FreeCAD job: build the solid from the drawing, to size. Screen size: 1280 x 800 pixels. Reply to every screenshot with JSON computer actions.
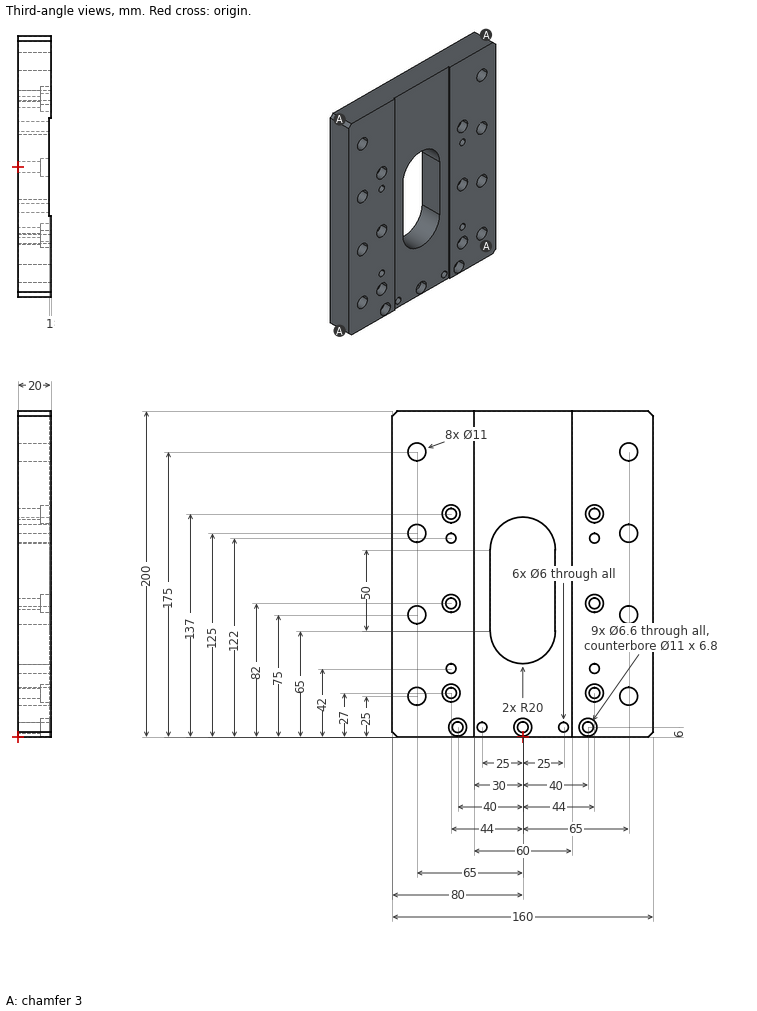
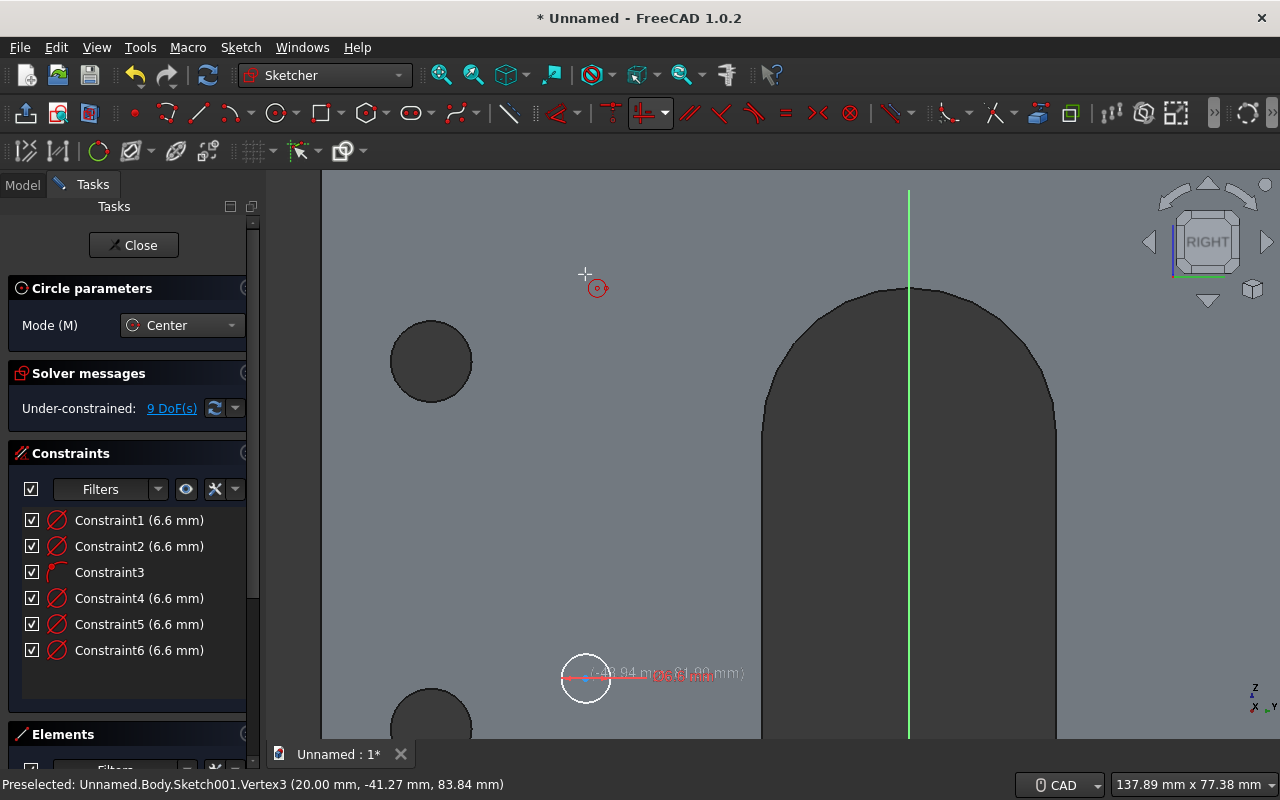
{"action": "left_click", "coordinate": [586, 273]}
{"action": "mouse_move", "coordinate": [603, 256]}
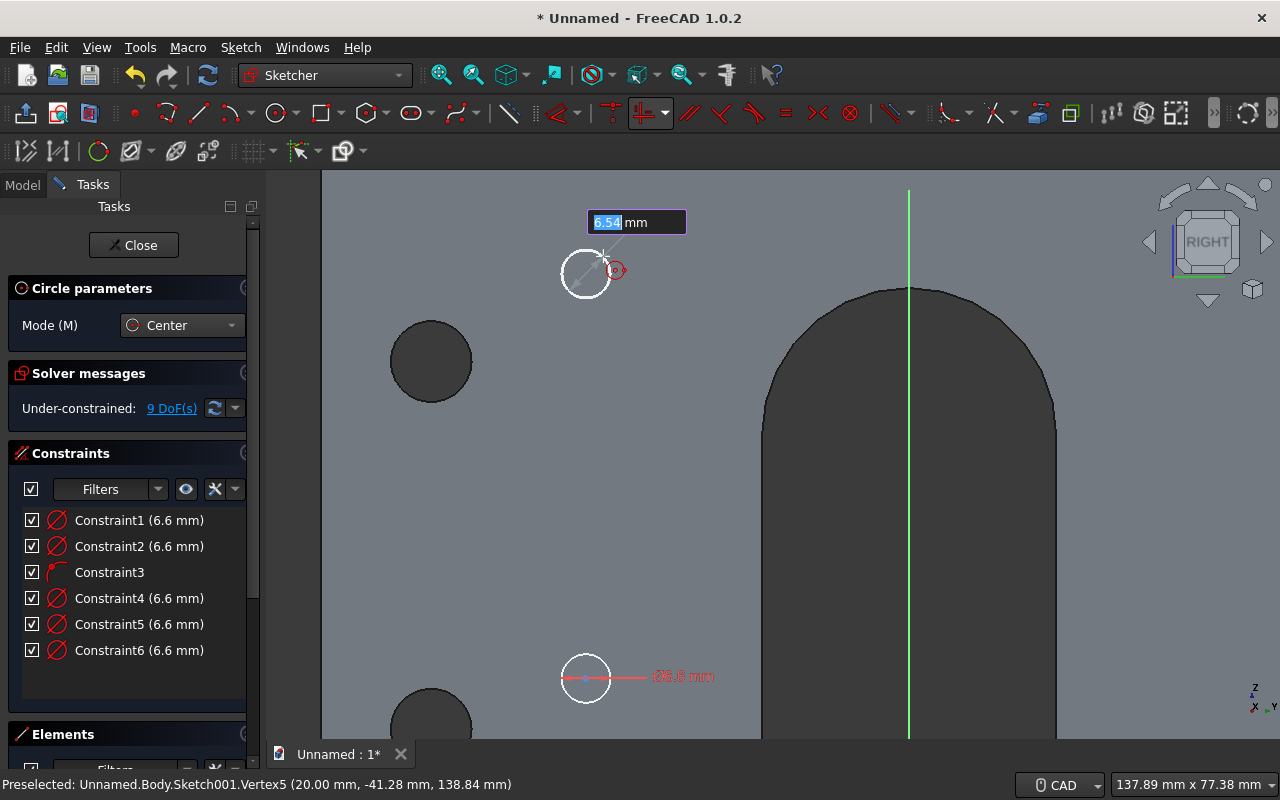
{"action": "type", "text": "6.6"}
{"action": "key", "text": "Return"}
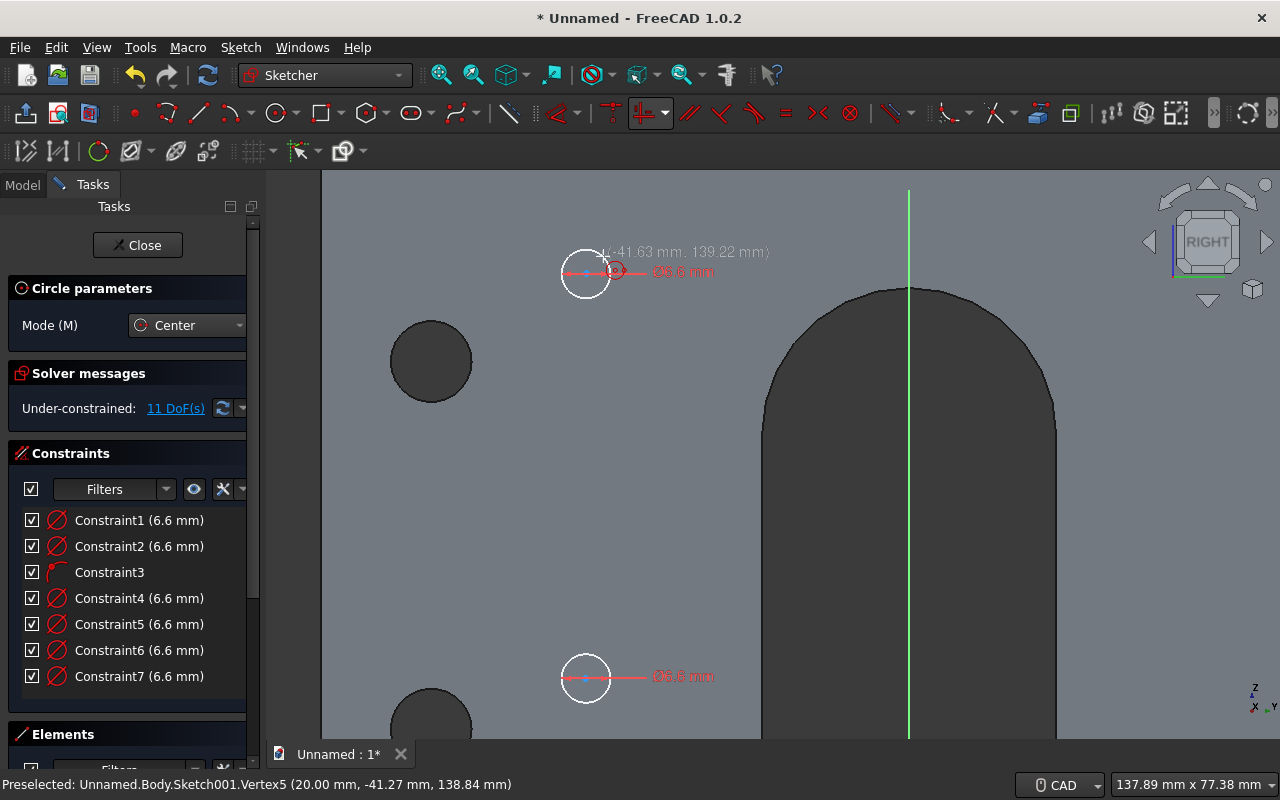
{"action": "scroll", "coordinate": [585, 274], "scroll_direction": "down", "scroll_amount": 5}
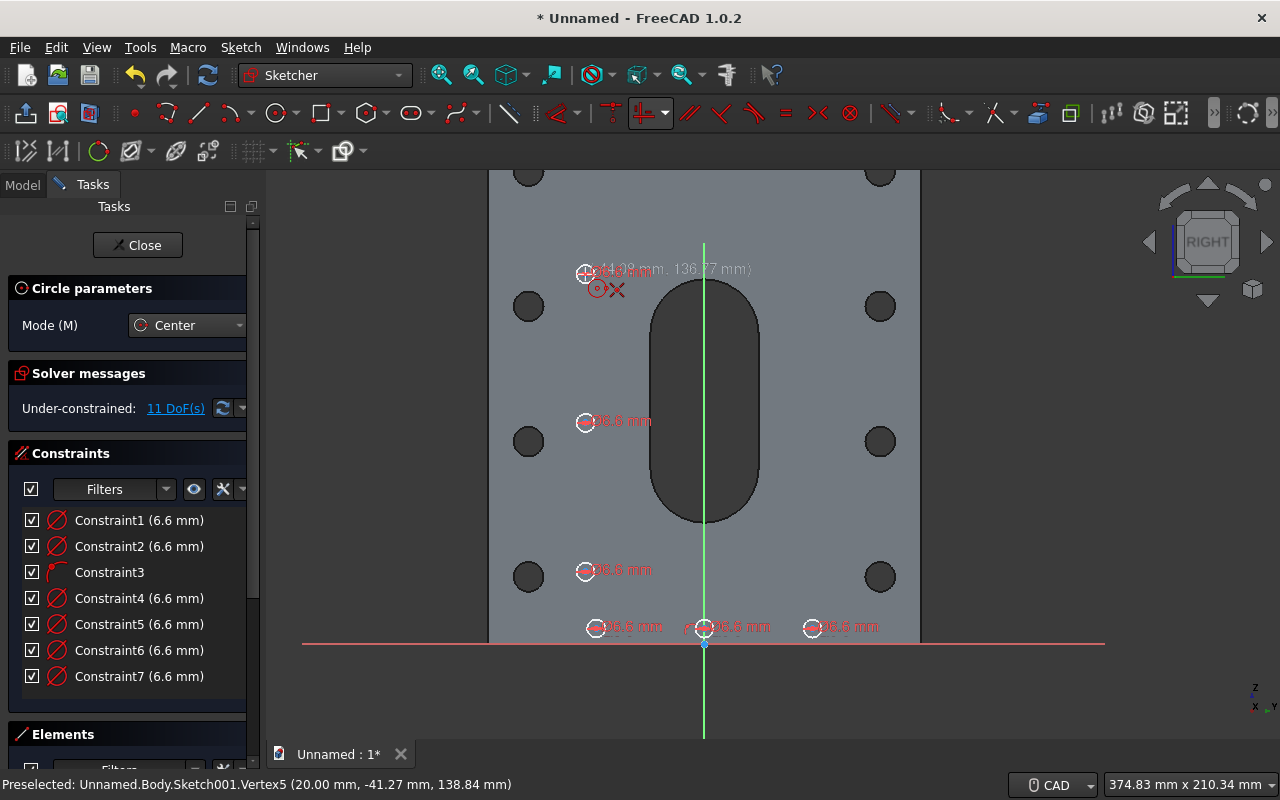
{"action": "scroll", "coordinate": [823, 571], "scroll_direction": "up", "scroll_amount": 5}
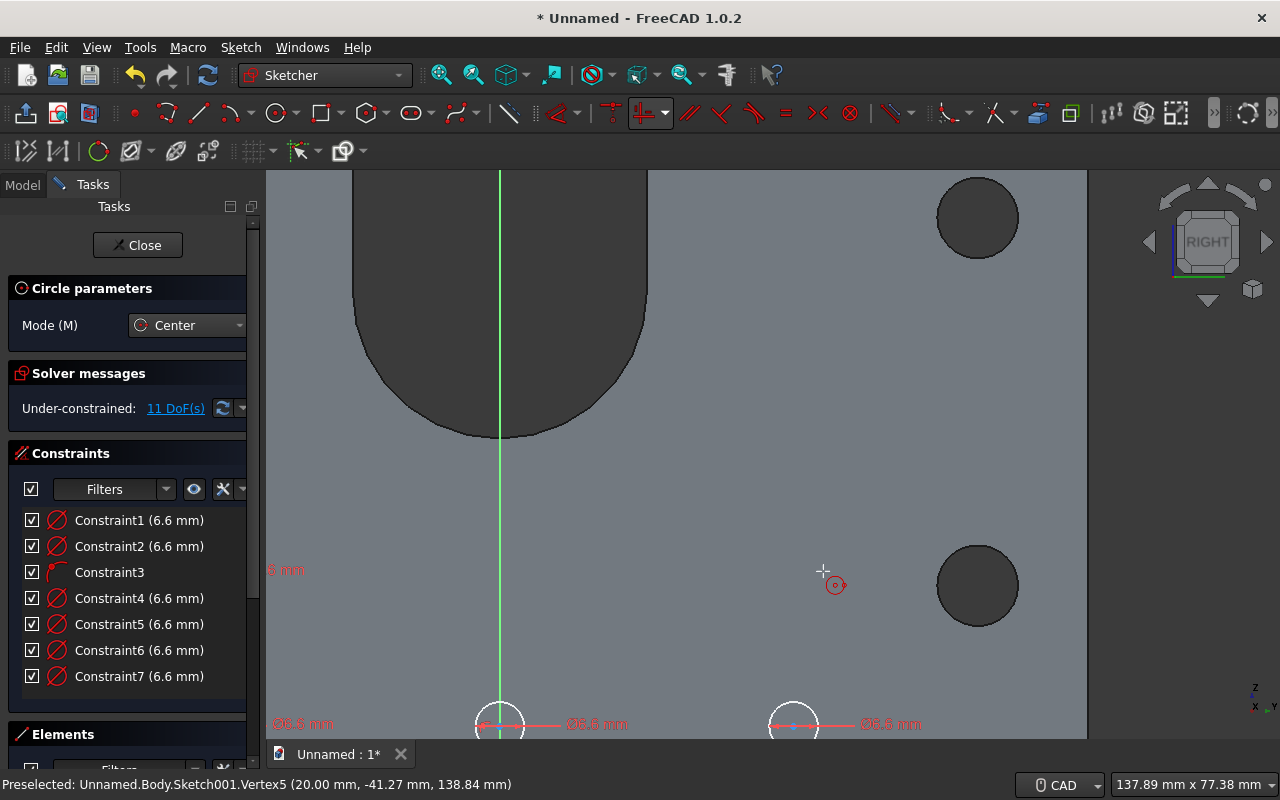
{"action": "left_click", "coordinate": [823, 571]}
{"action": "mouse_move", "coordinate": [840, 554]}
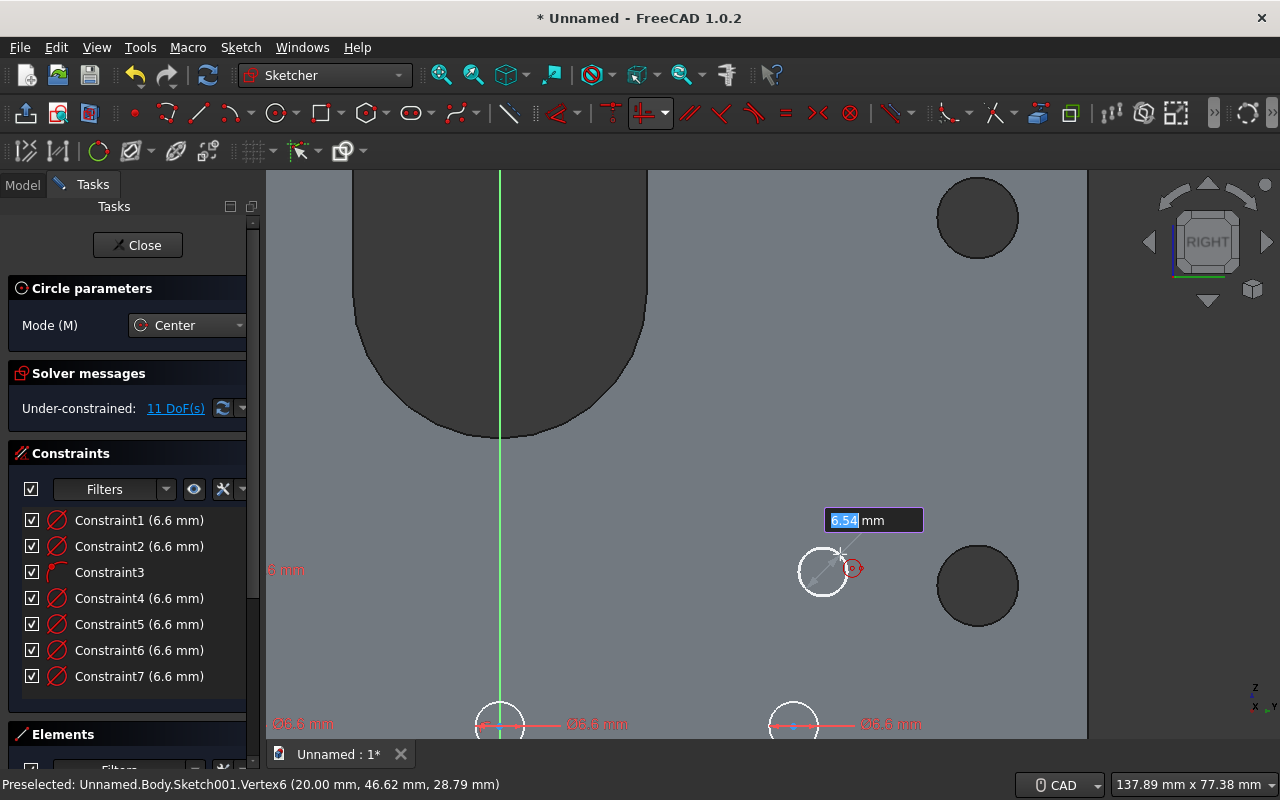
{"action": "type", "text": "6.6"}
{"action": "key", "text": "Return"}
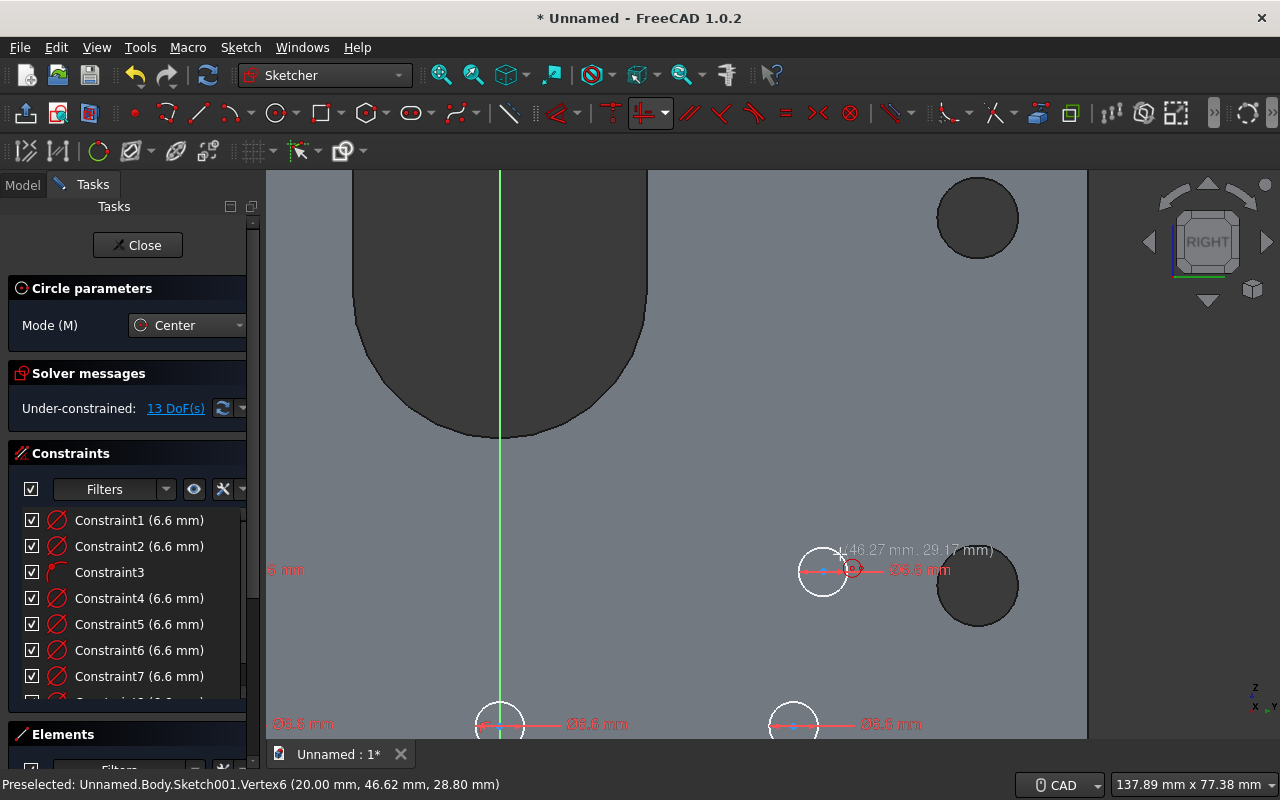
{"action": "scroll", "coordinate": [824, 571], "scroll_direction": "down", "scroll_amount": 5}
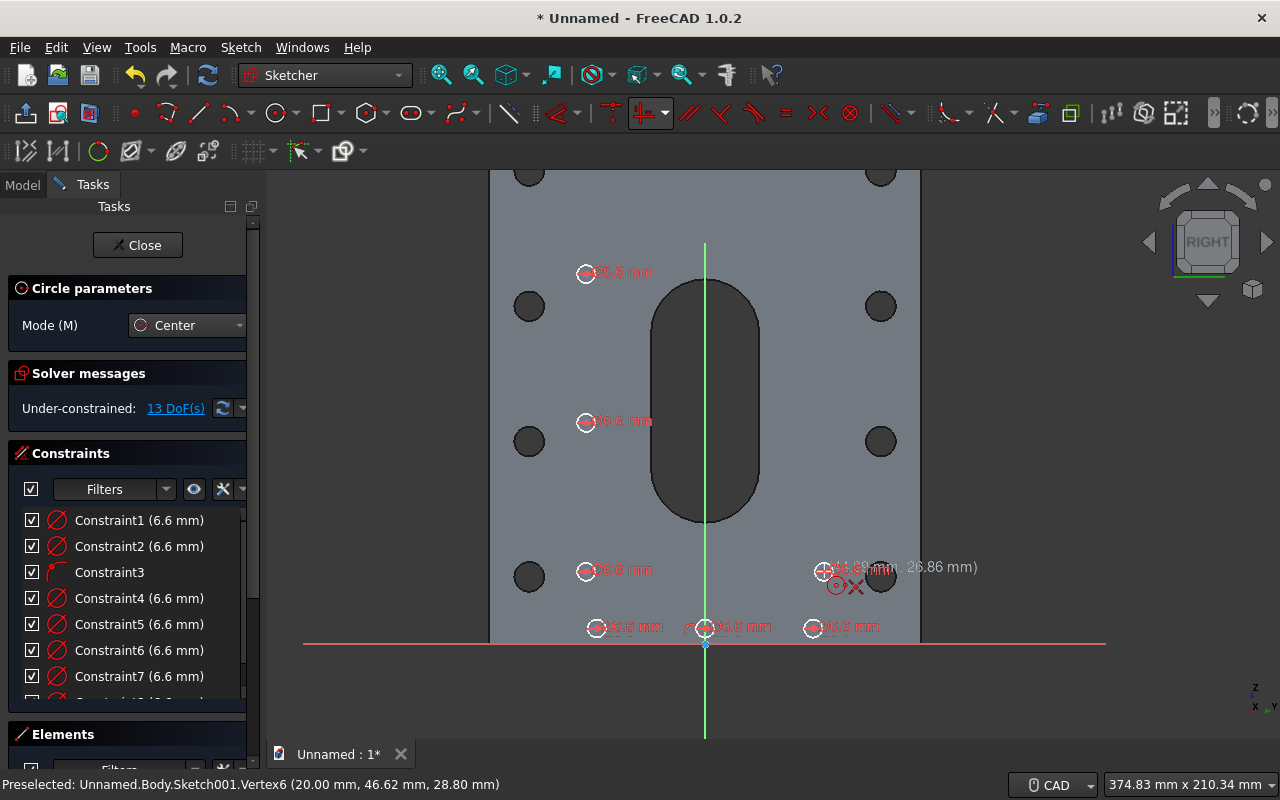
{"action": "scroll", "coordinate": [824, 423], "scroll_direction": "up", "scroll_amount": 5}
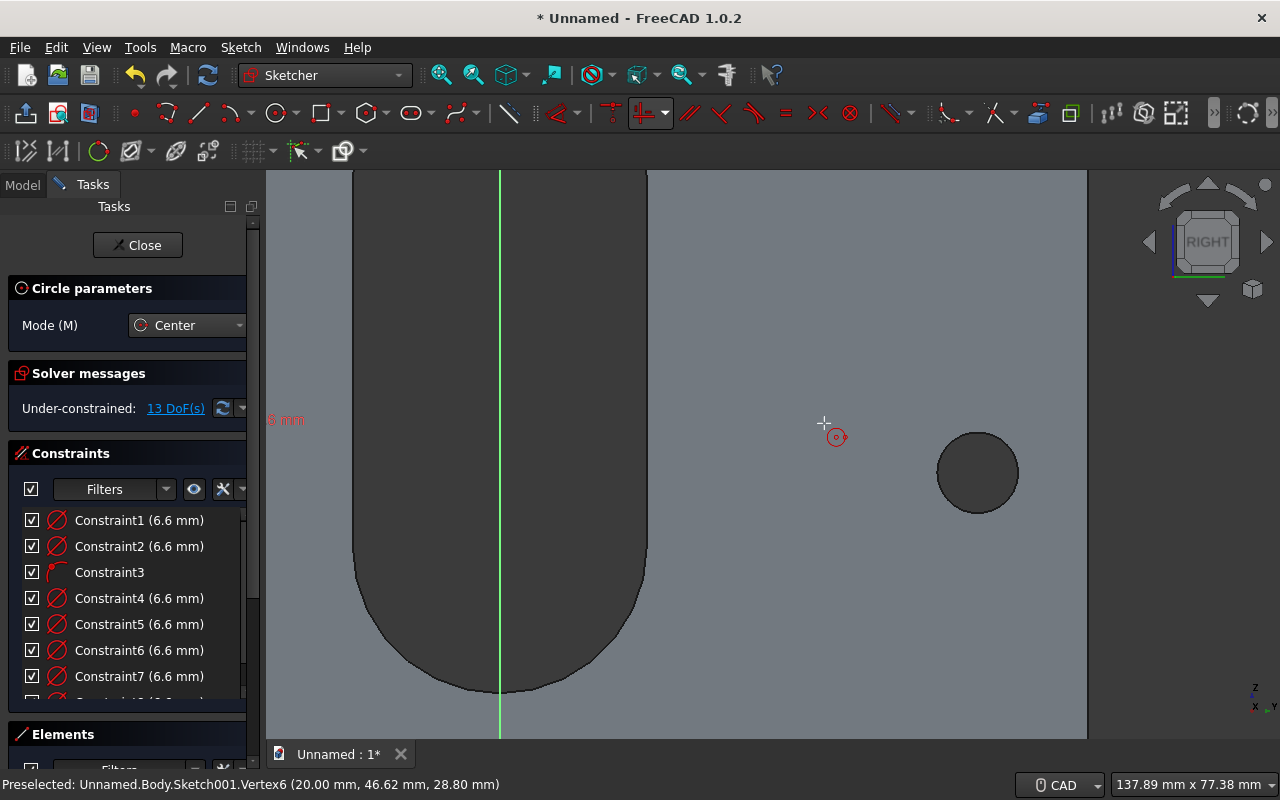
{"action": "left_click", "coordinate": [823, 421]}
{"action": "mouse_move", "coordinate": [840, 404]}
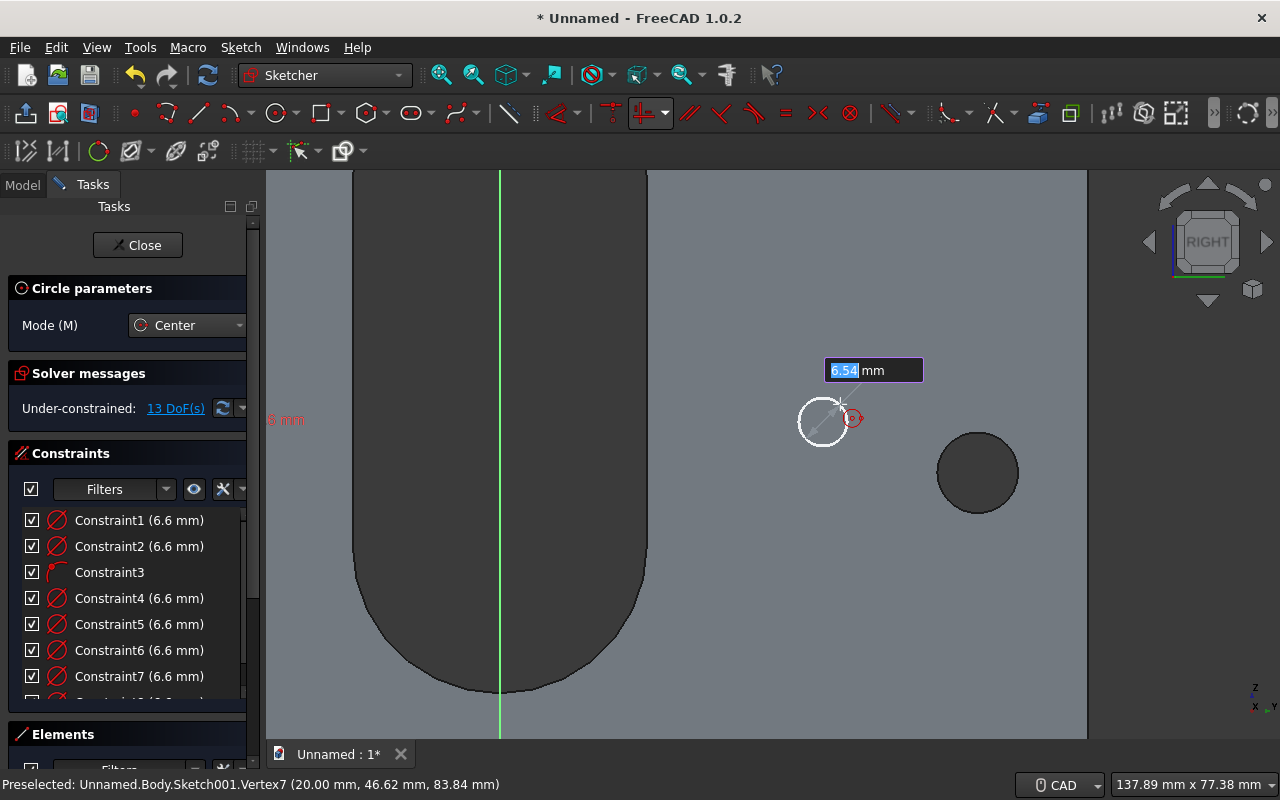
{"action": "type", "text": "6.6"}
{"action": "key", "text": "Return"}